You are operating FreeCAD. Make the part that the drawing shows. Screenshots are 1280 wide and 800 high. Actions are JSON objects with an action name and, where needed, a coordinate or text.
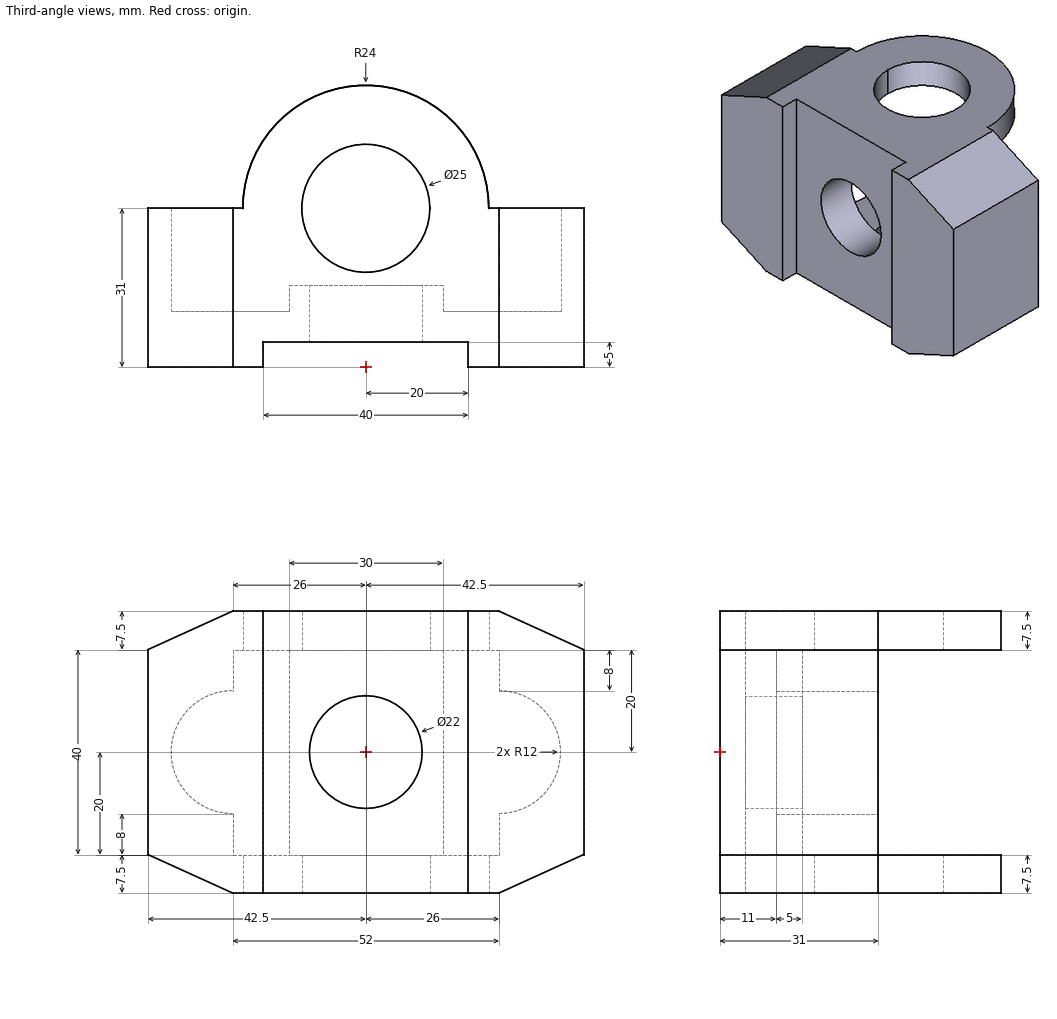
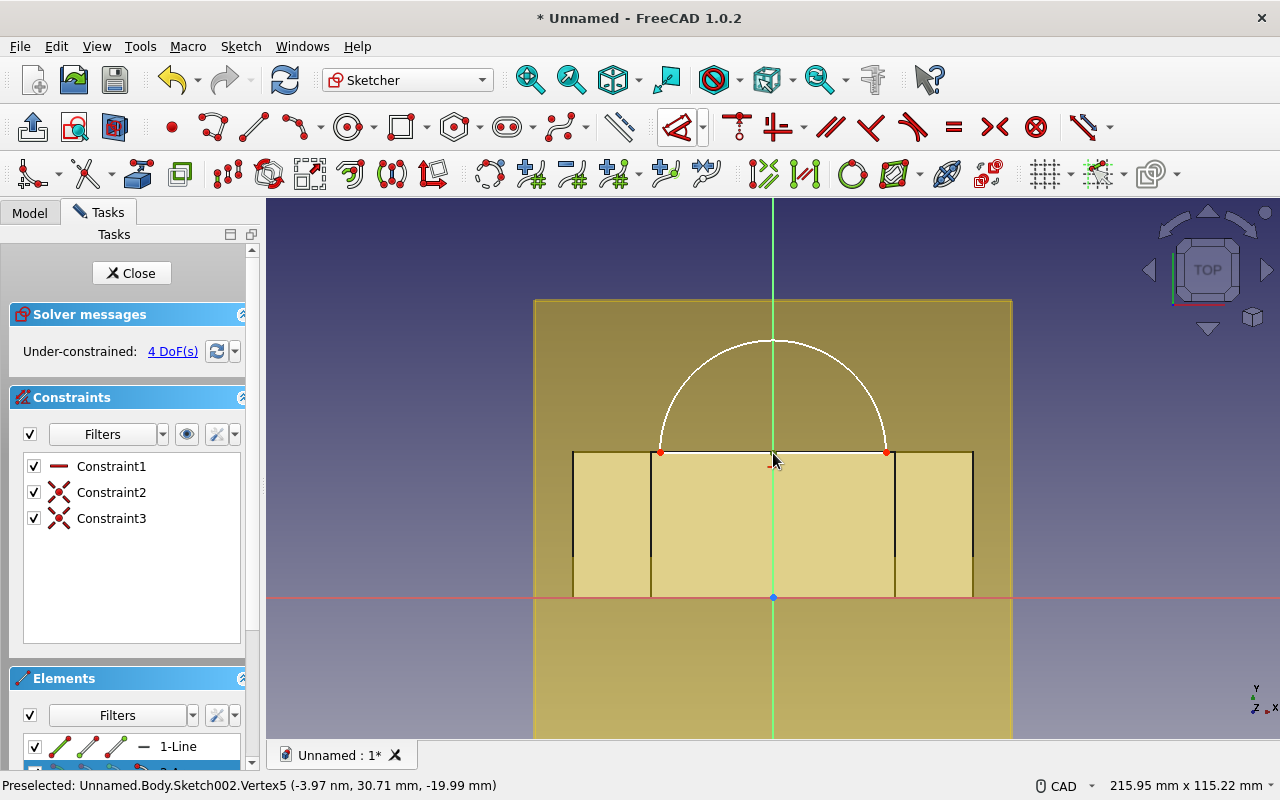
{"action": "left_click", "coordinate": [773, 676]}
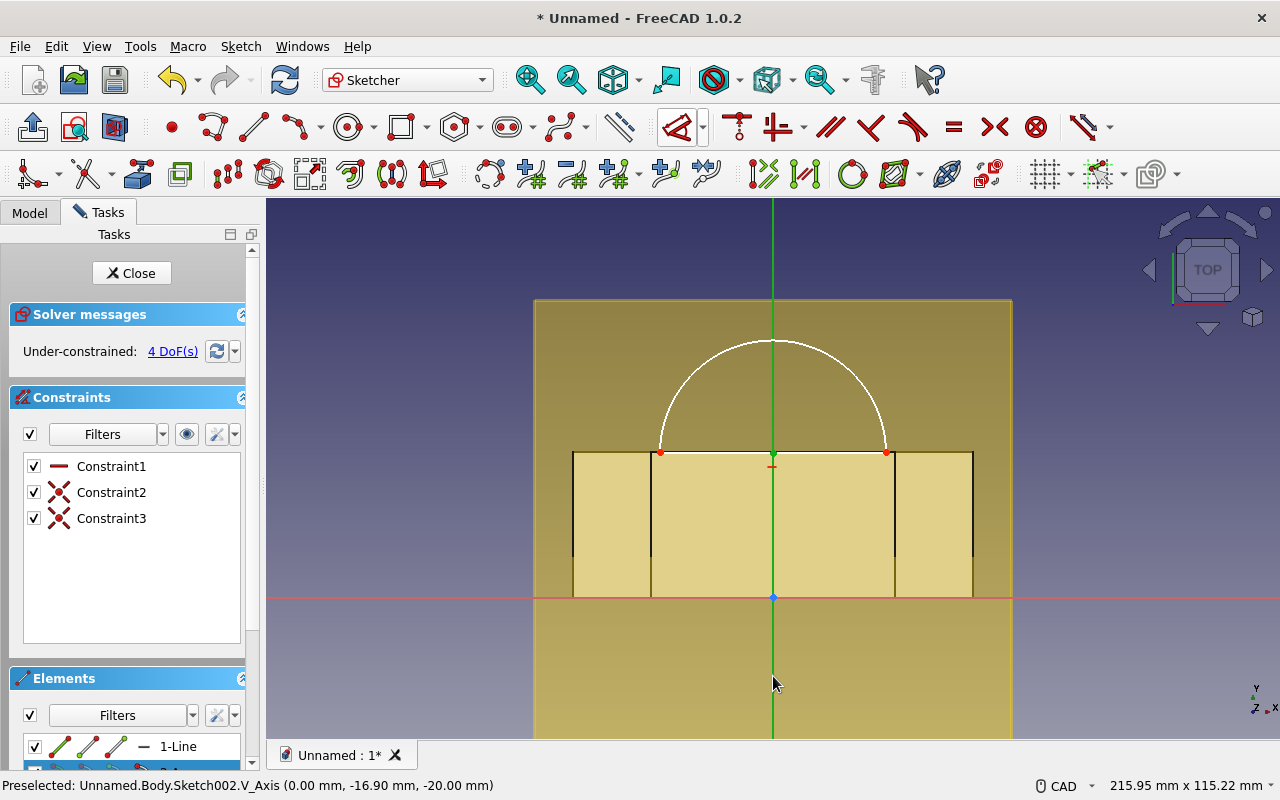
{"action": "left_click", "coordinate": [737, 128]}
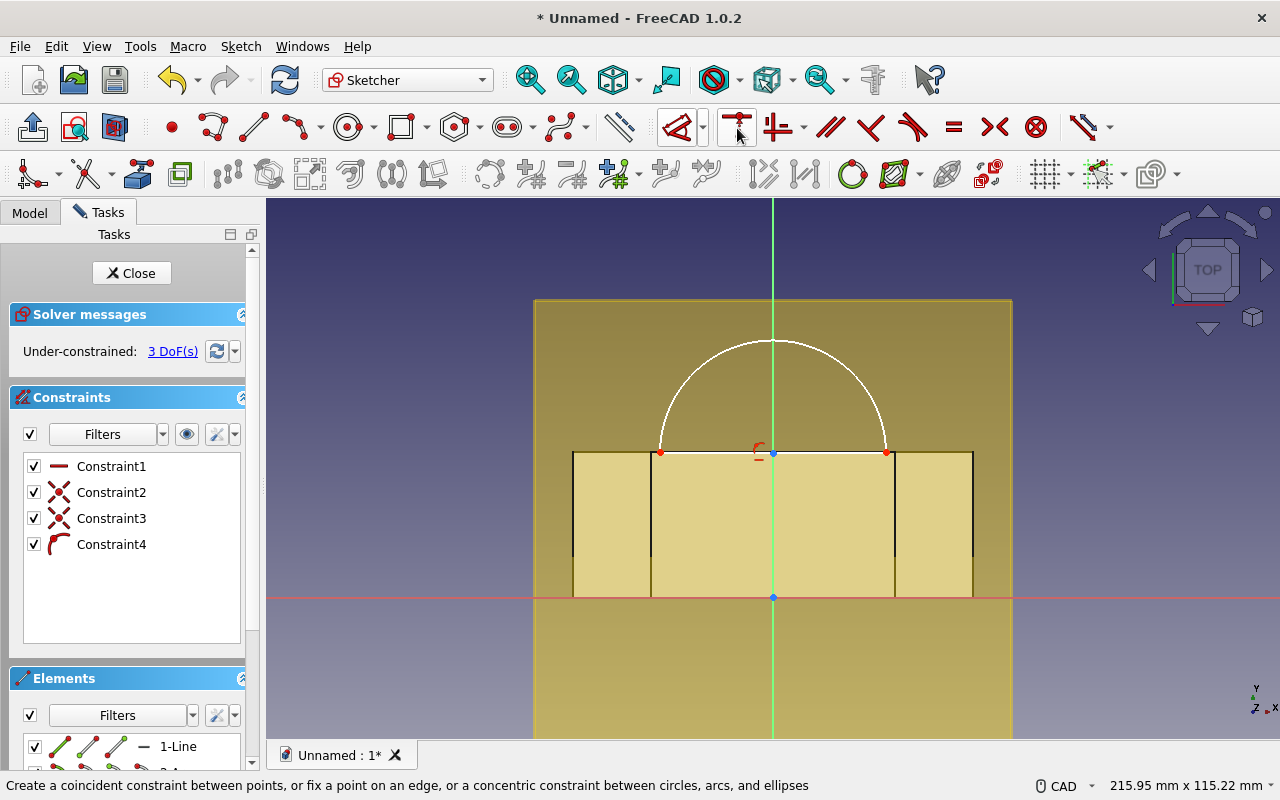
{"action": "left_click", "coordinate": [839, 362]}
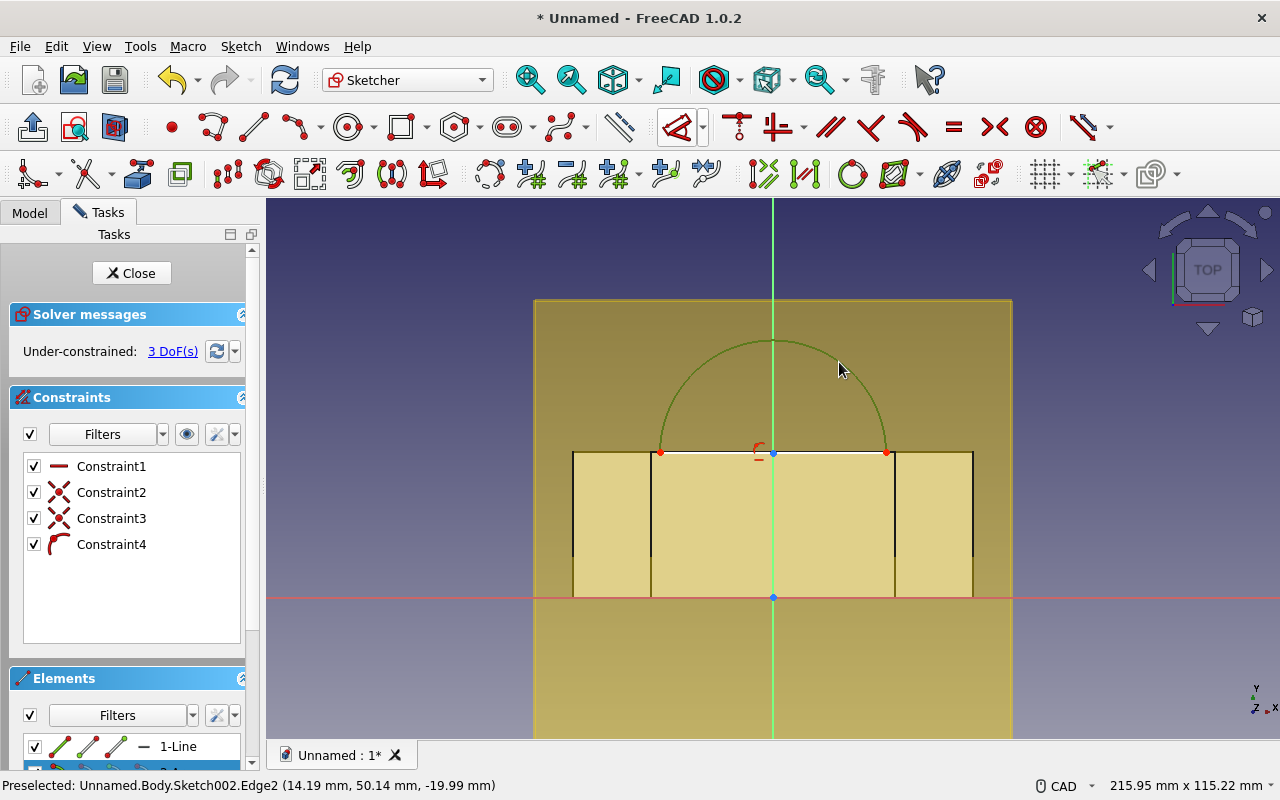
{"action": "left_click", "coordinate": [702, 128]}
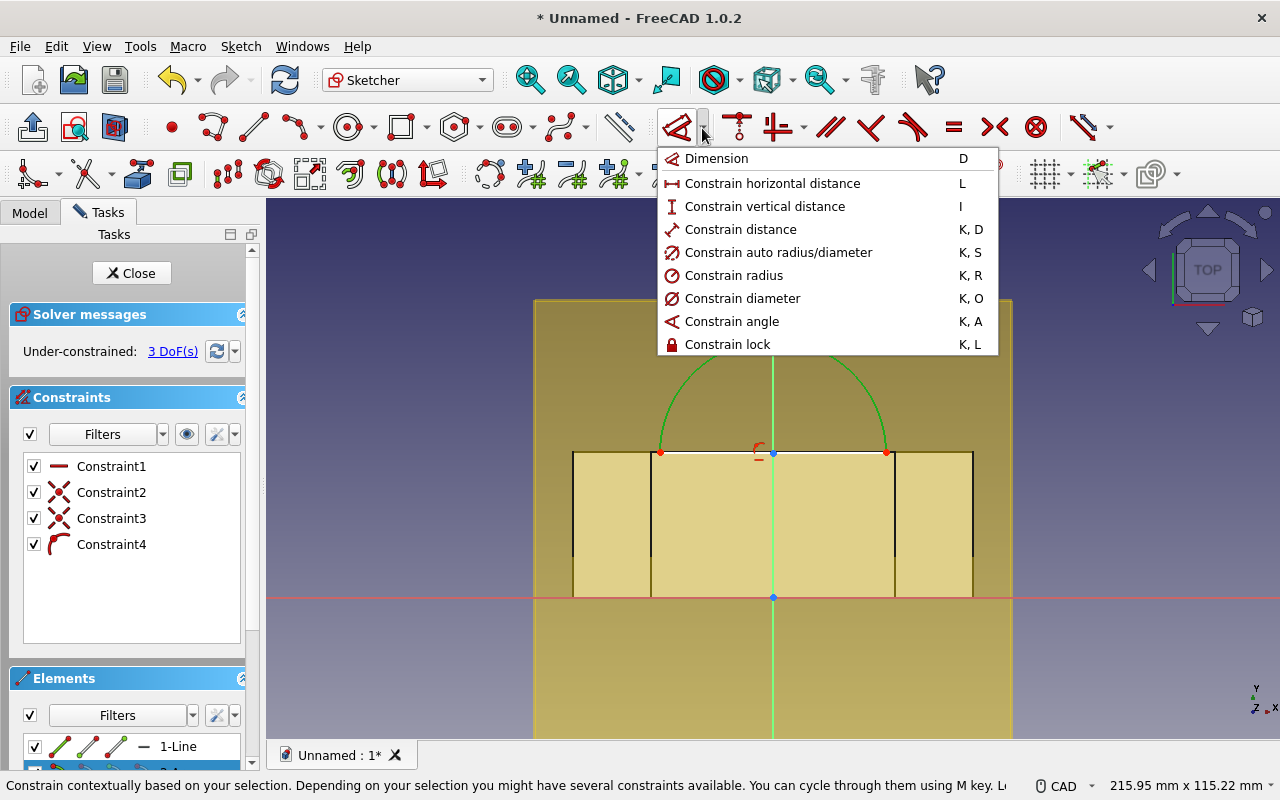
{"action": "left_click", "coordinate": [828, 276]}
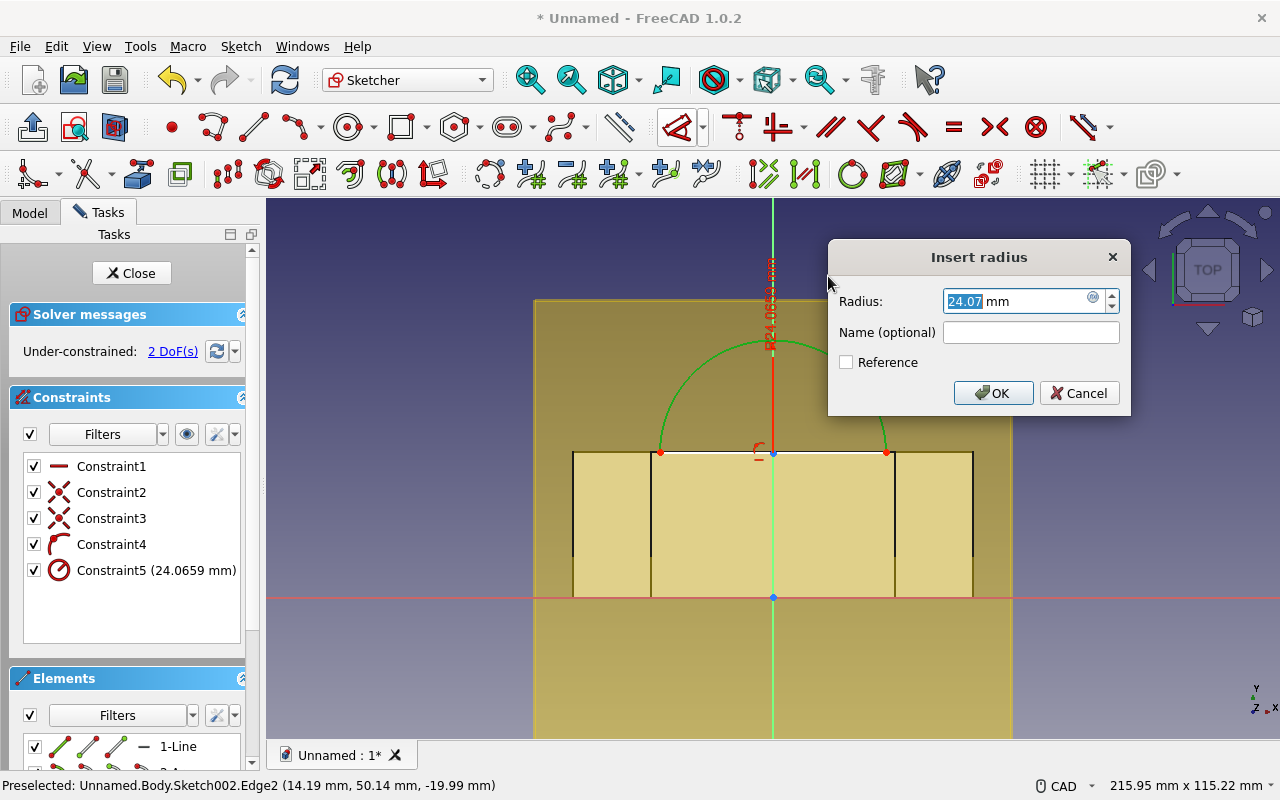
{"action": "type", "text": "24"}
{"action": "key", "text": "Return"}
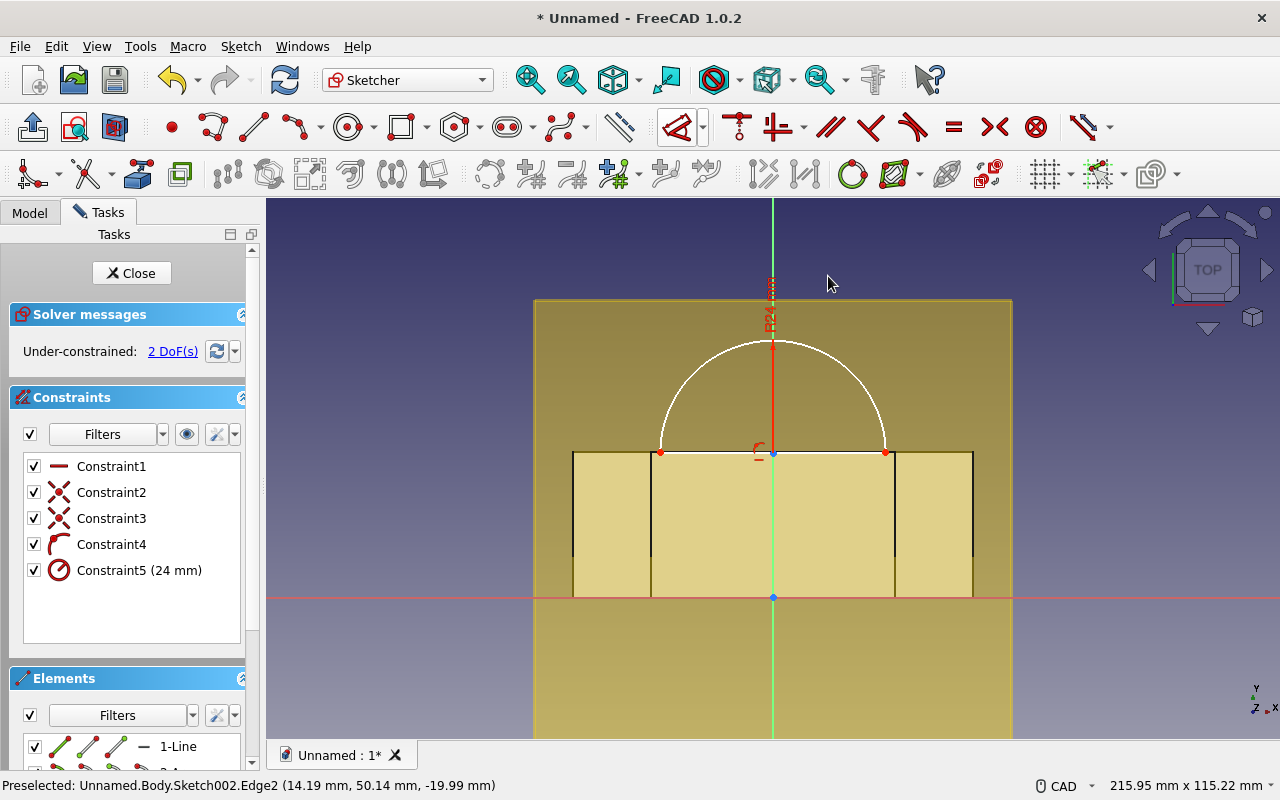
{"action": "left_click", "coordinate": [886, 453]}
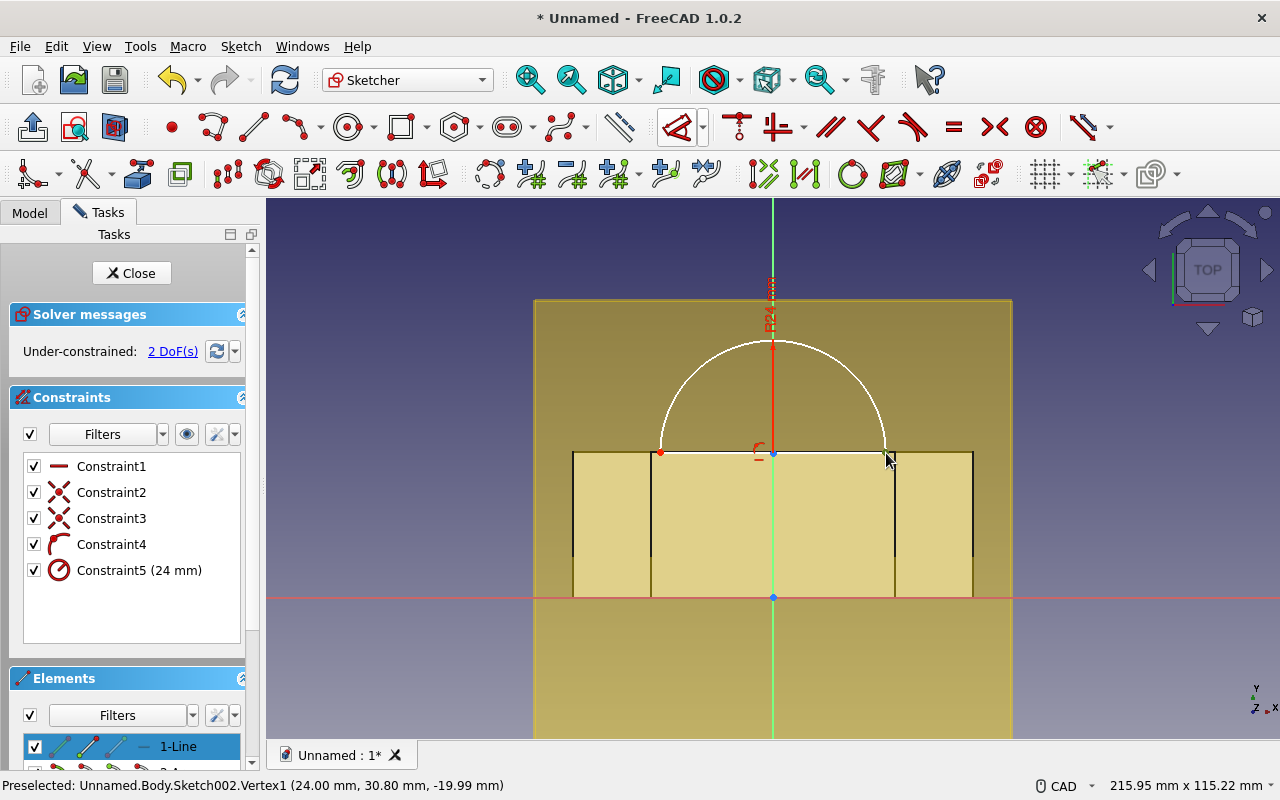
{"action": "left_click", "coordinate": [702, 128]}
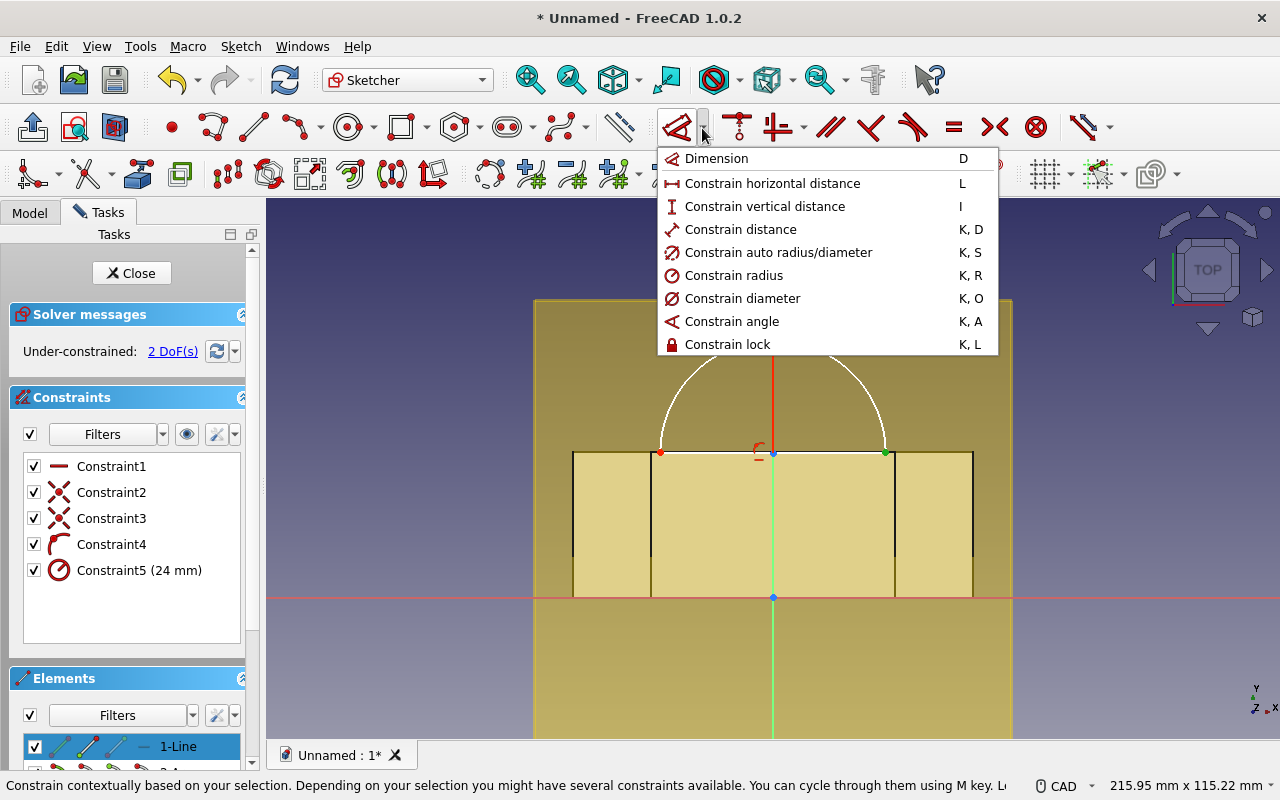
{"action": "left_click", "coordinate": [828, 206]}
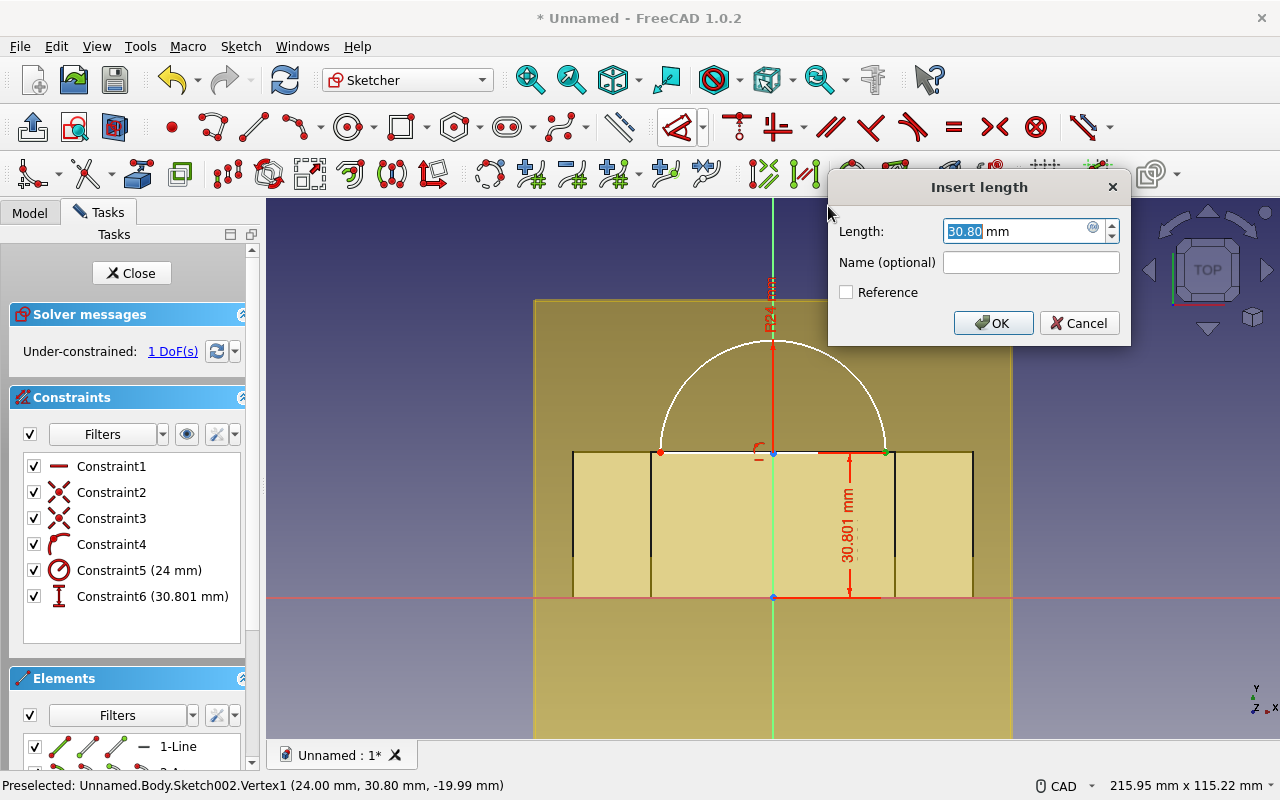
{"action": "type", "text": "31"}
{"action": "key", "text": "Return"}